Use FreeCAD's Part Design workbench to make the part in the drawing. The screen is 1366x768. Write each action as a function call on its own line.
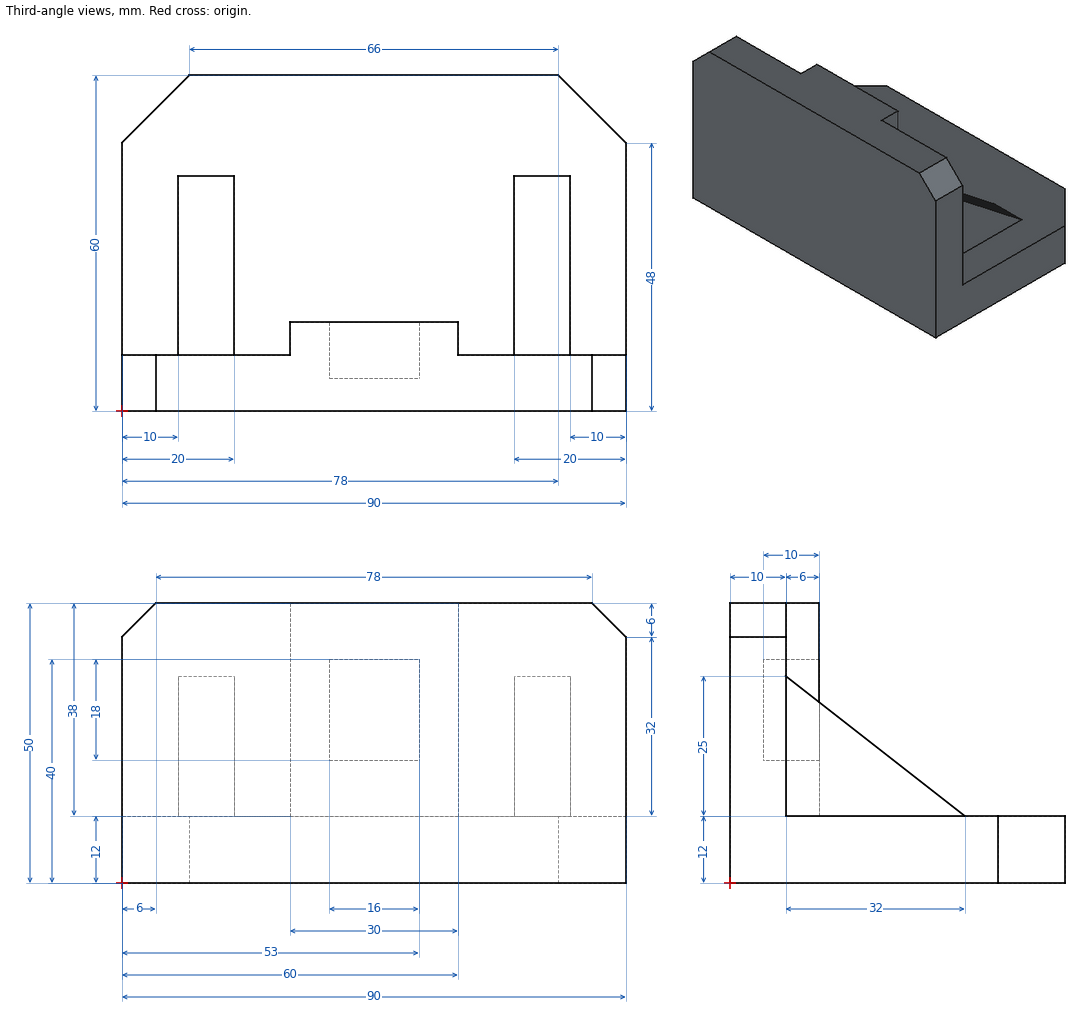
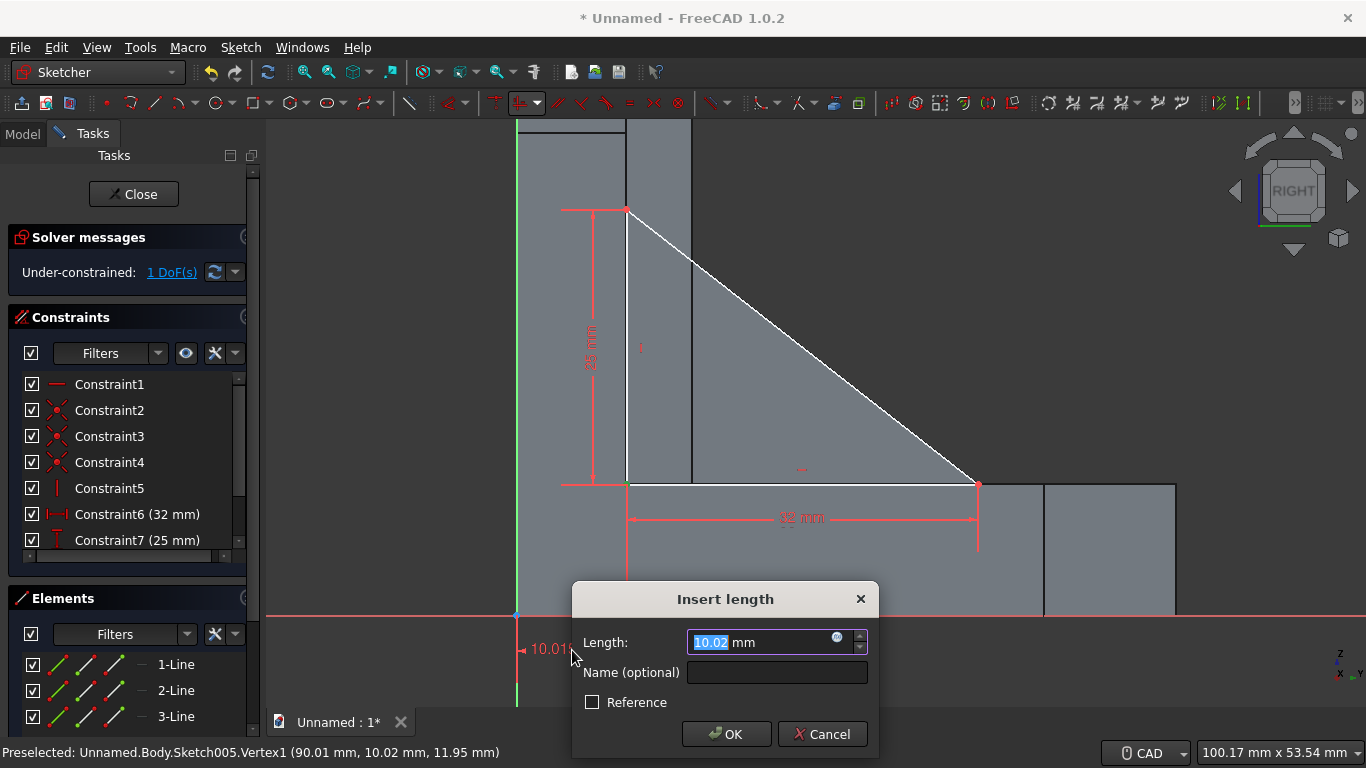
text(10)
key(Return)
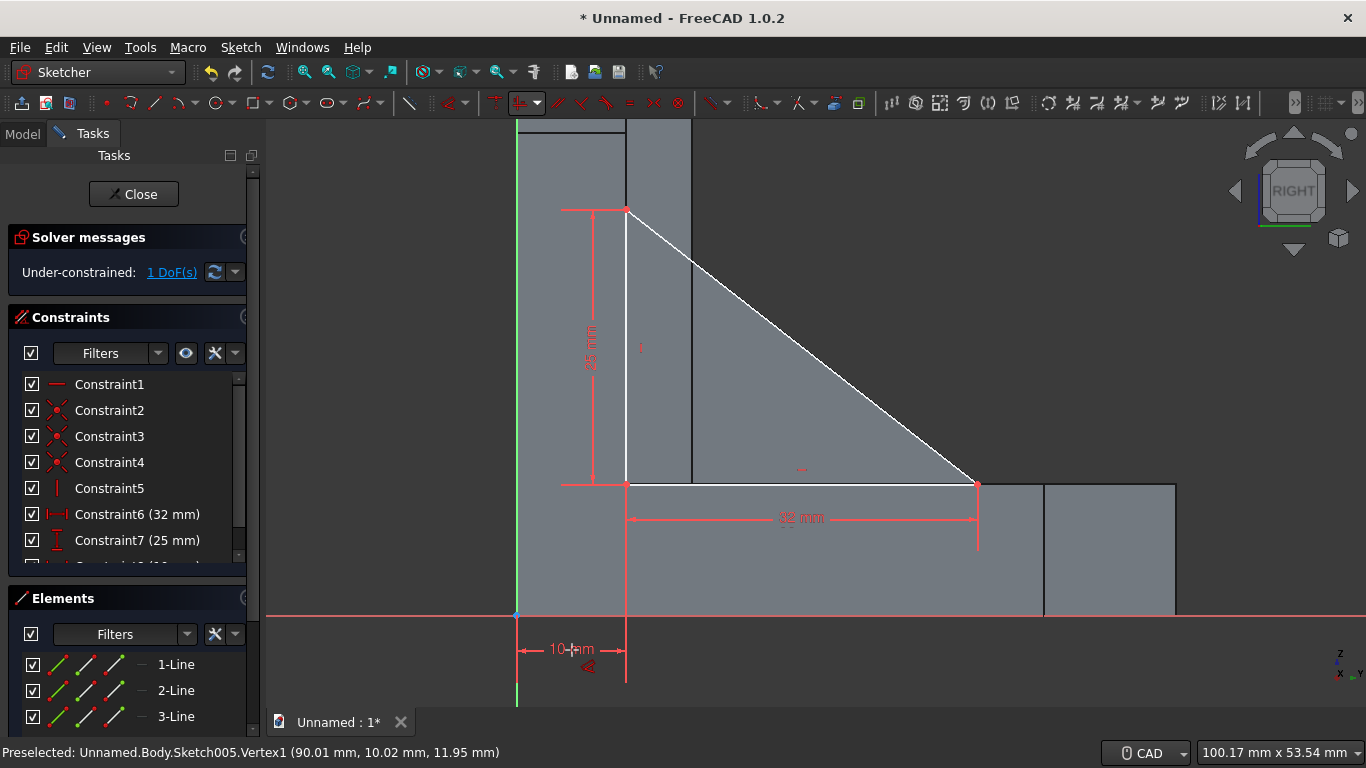
click(626, 485)
click(483, 550)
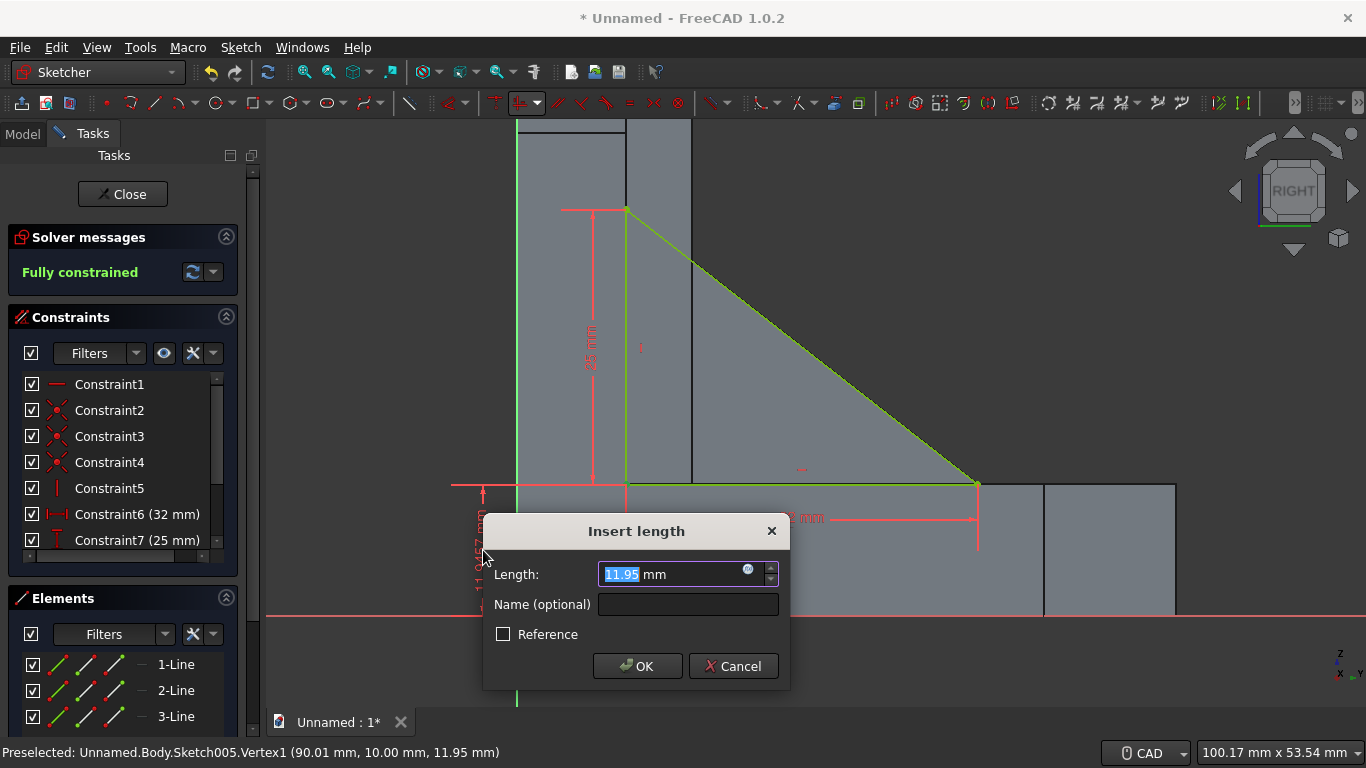
text(12)
key(Return)
key(Escape)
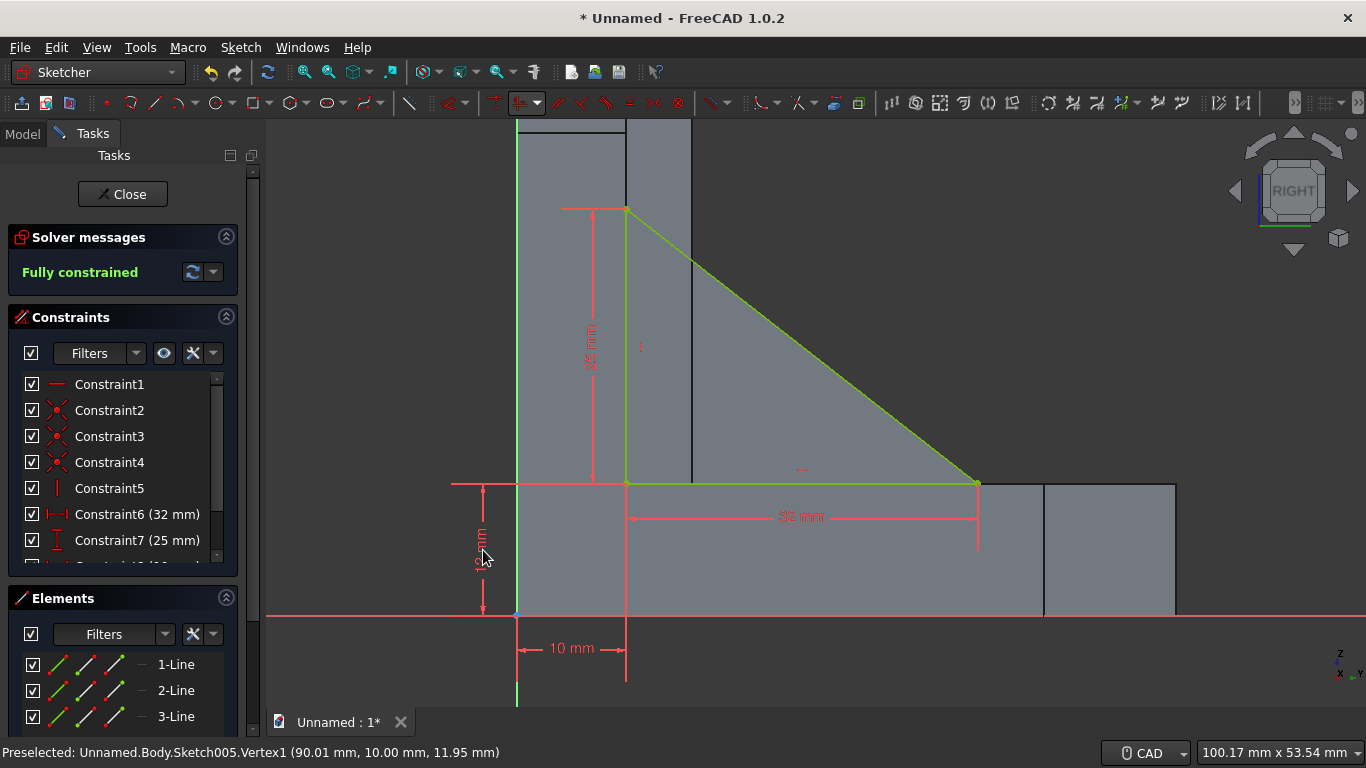
click(123, 194)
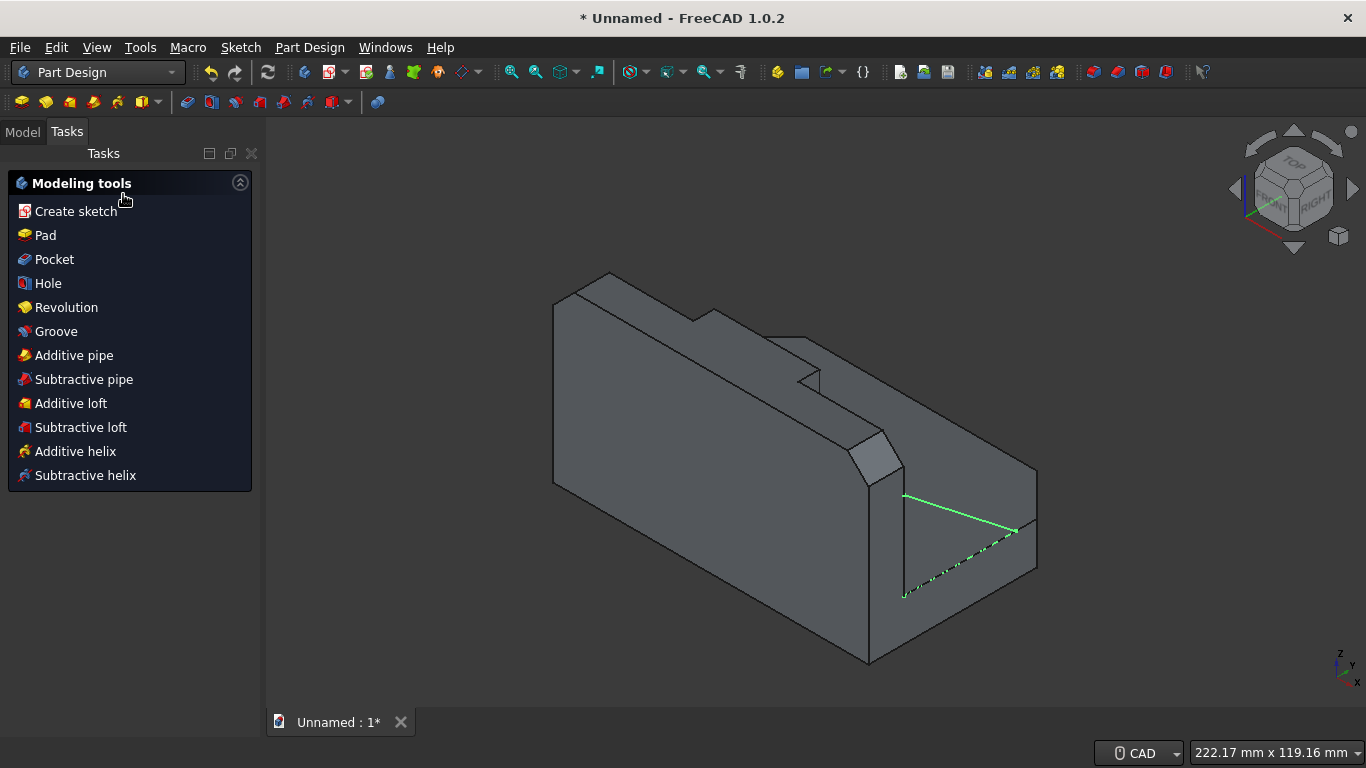
click(22, 102)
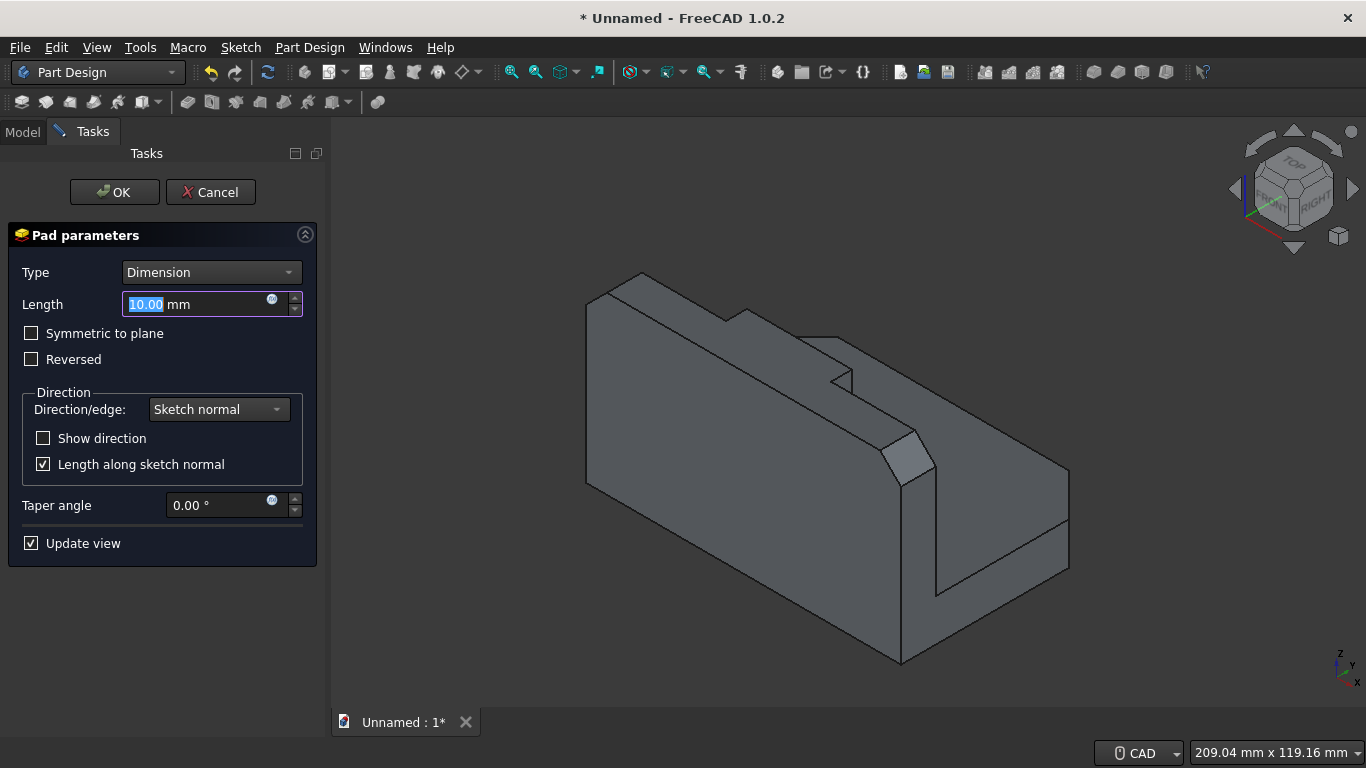
text(20)
key(Tab)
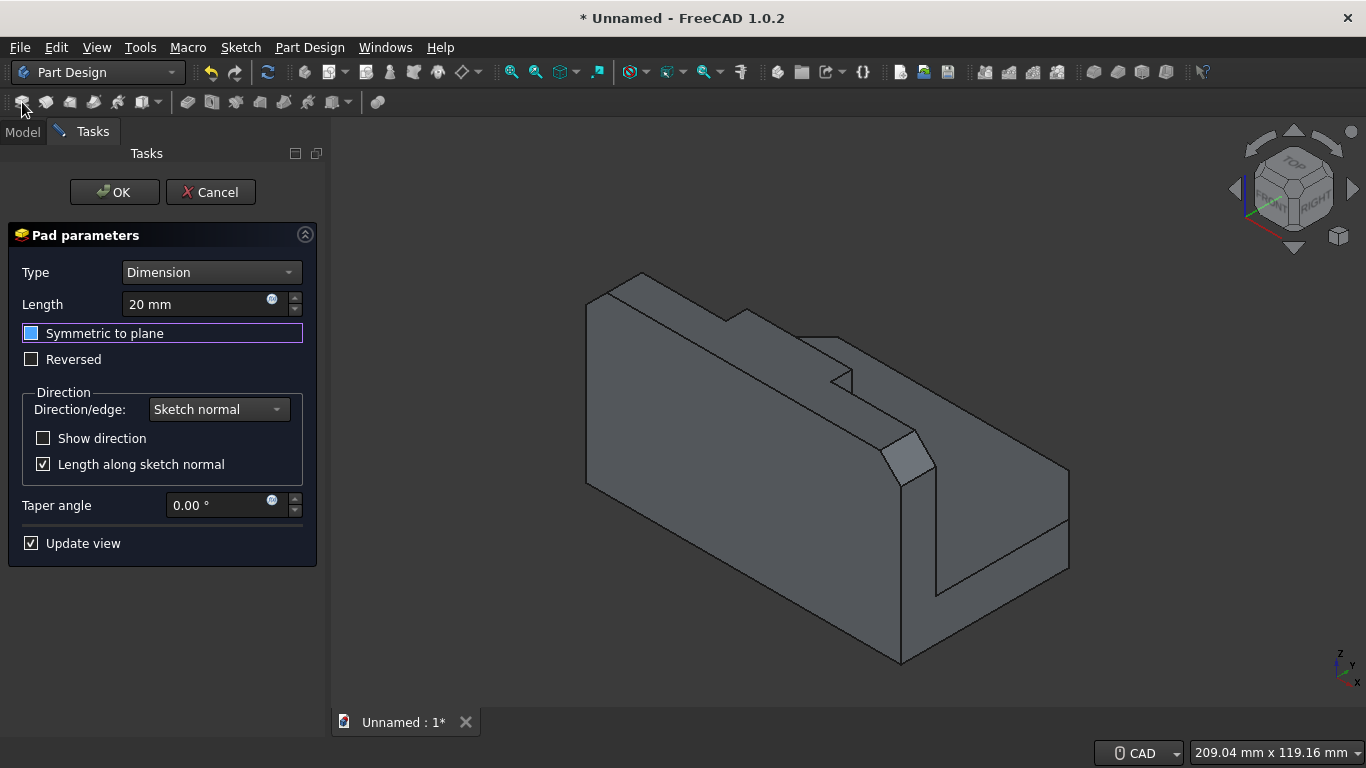
click(30, 359)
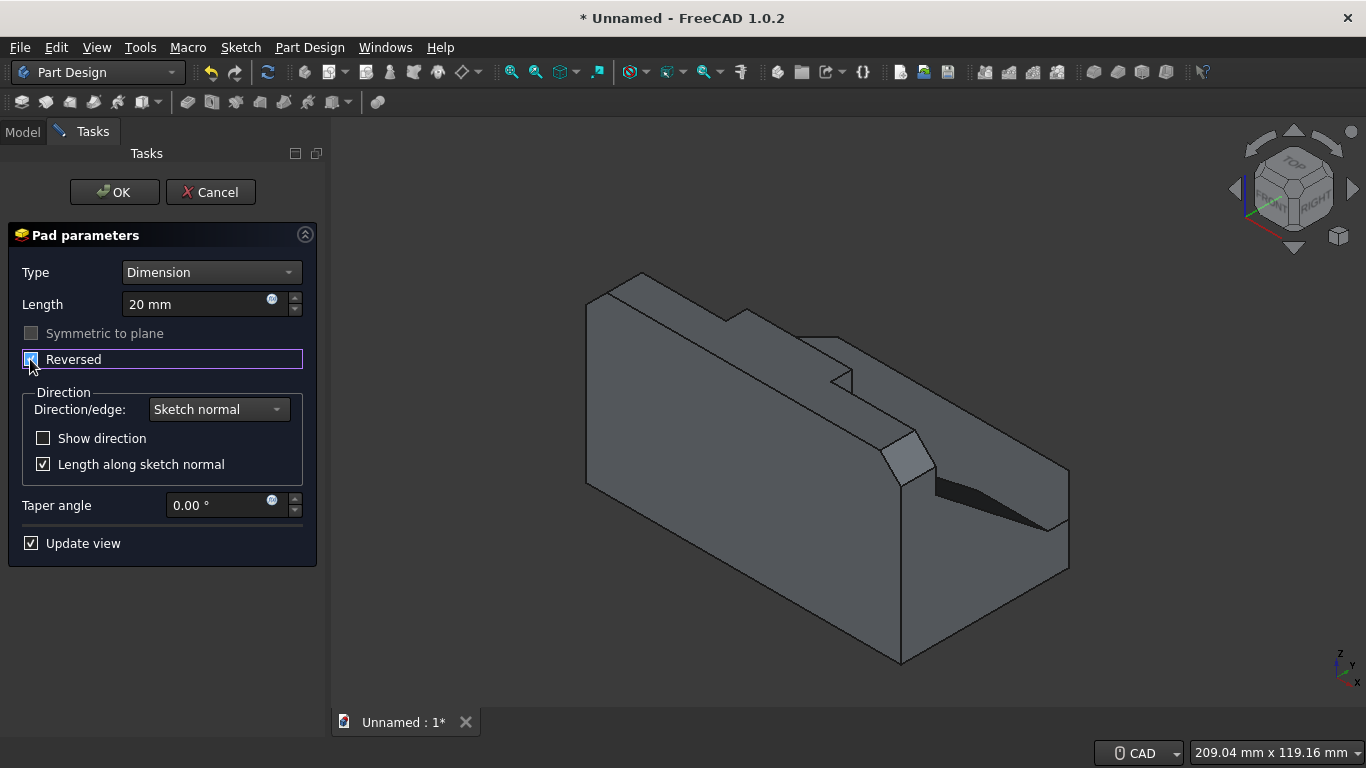
click(115, 192)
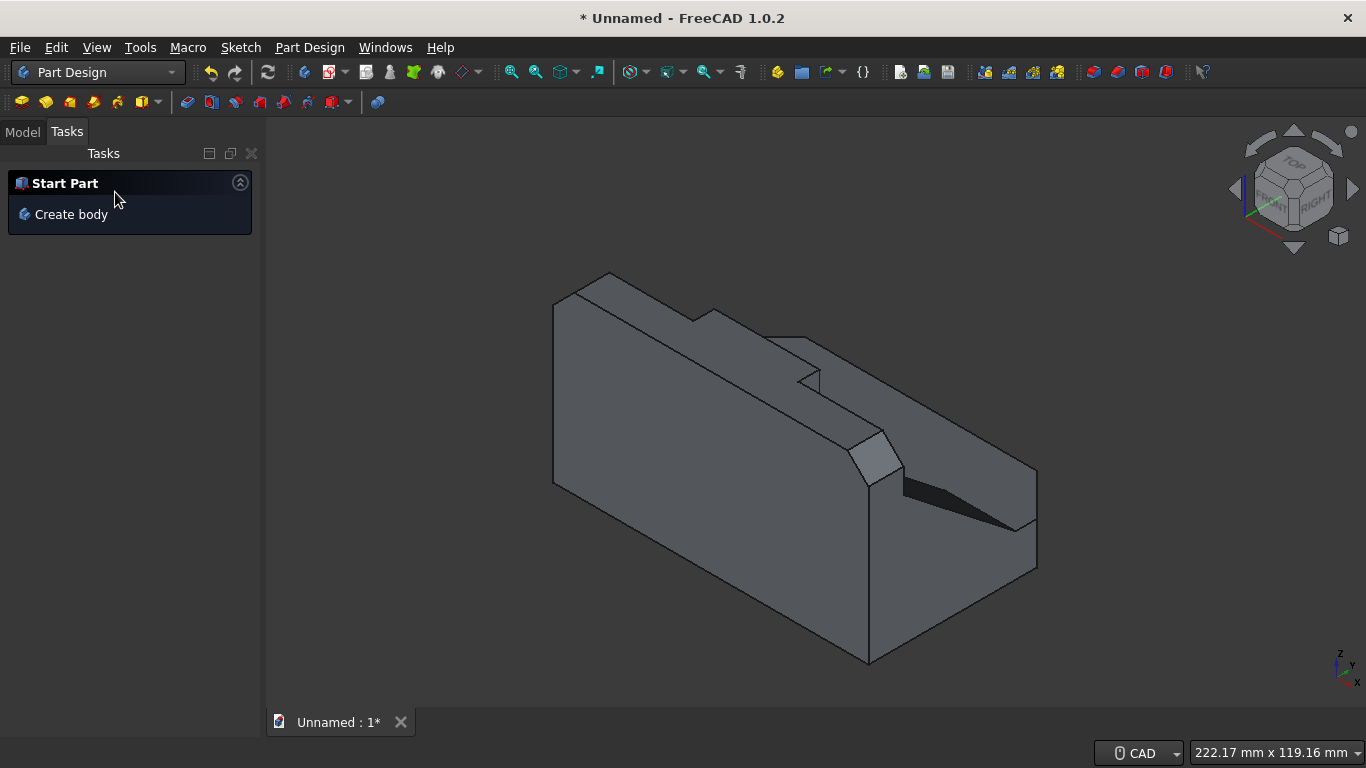
click(929, 565)